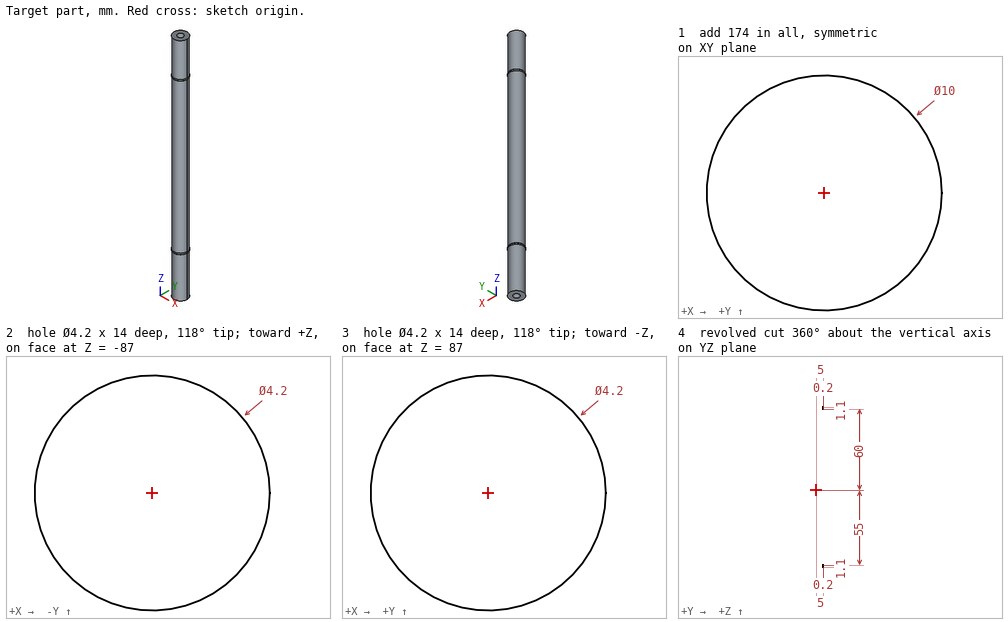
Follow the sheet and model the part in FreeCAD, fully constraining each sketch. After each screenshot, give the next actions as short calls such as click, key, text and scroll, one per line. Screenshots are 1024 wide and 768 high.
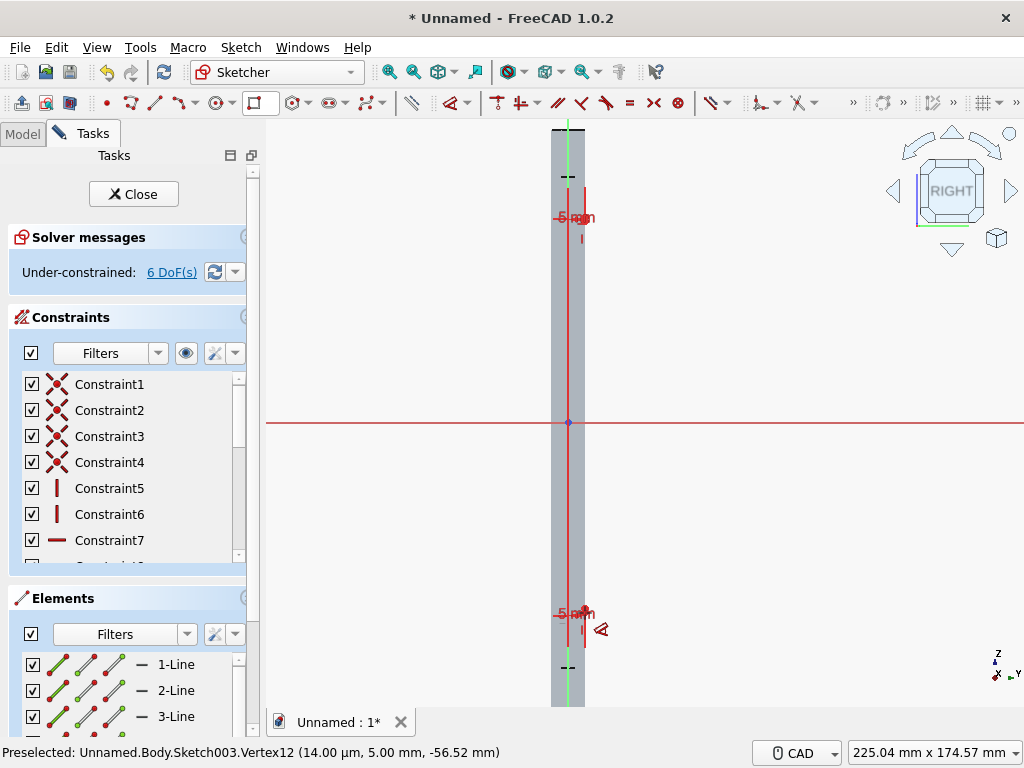
scroll(584, 219, up, 14)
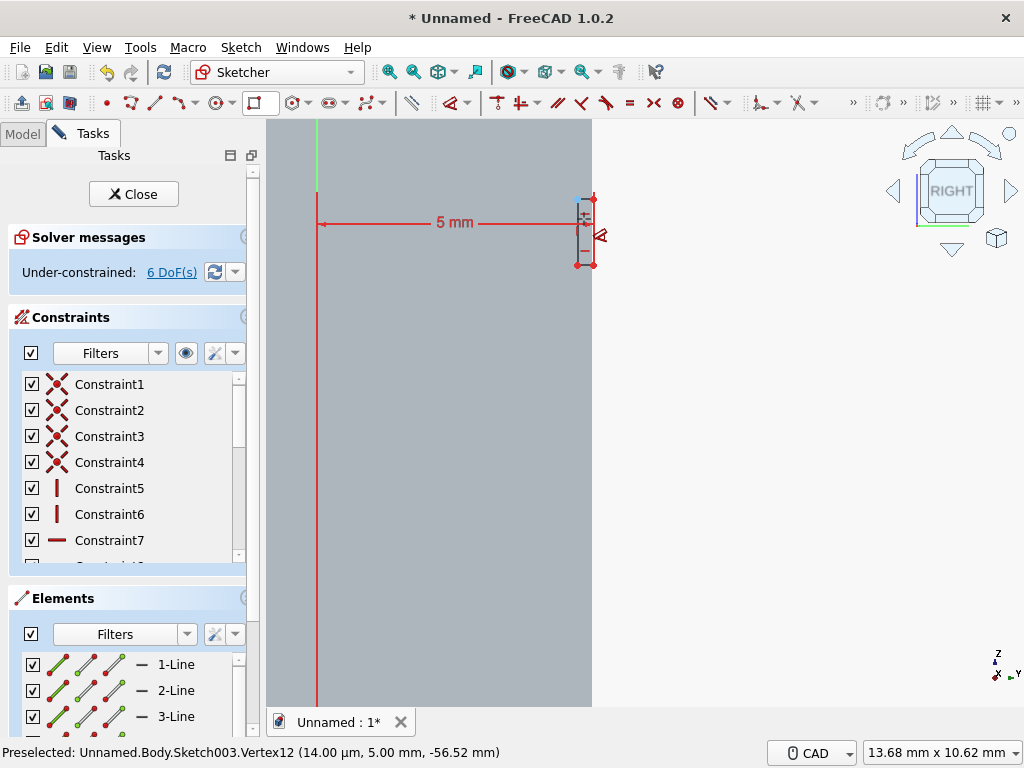
click(578, 219)
click(612, 232)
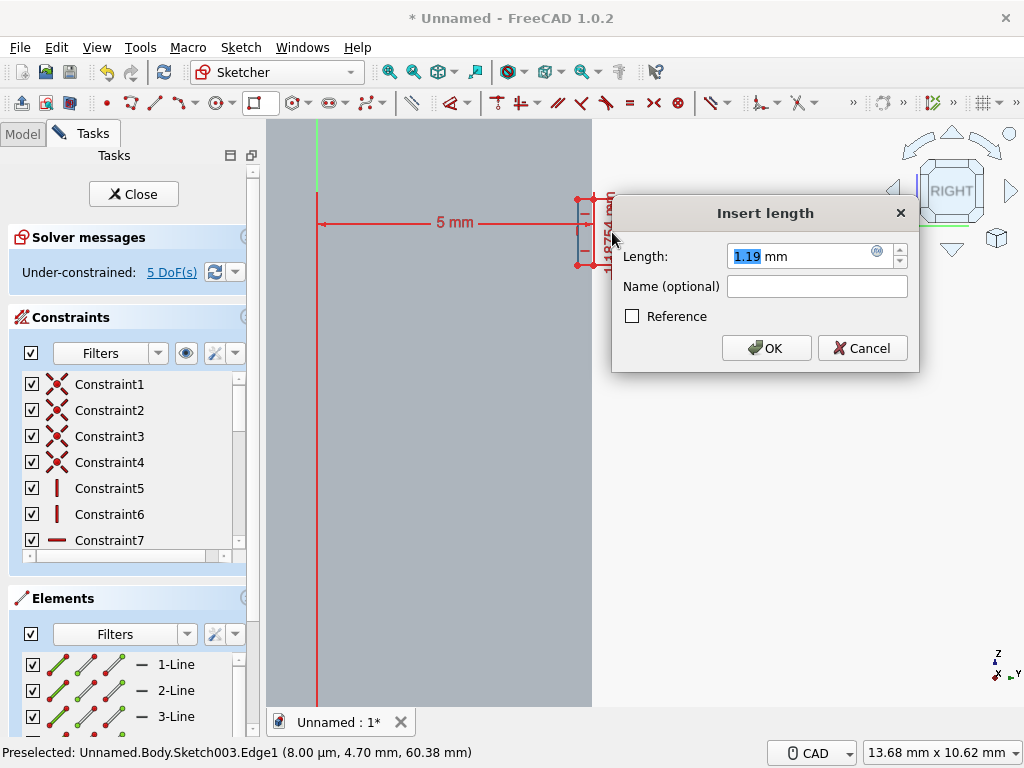
text(1.1)
key(Return)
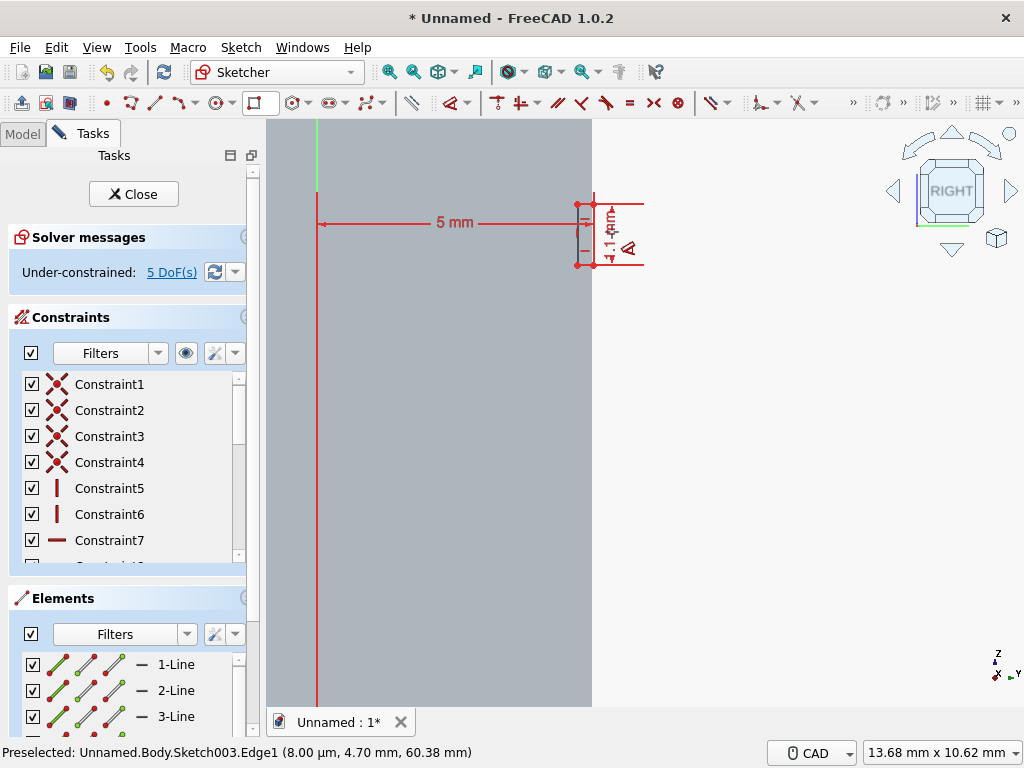
scroll(586, 265, up, 7)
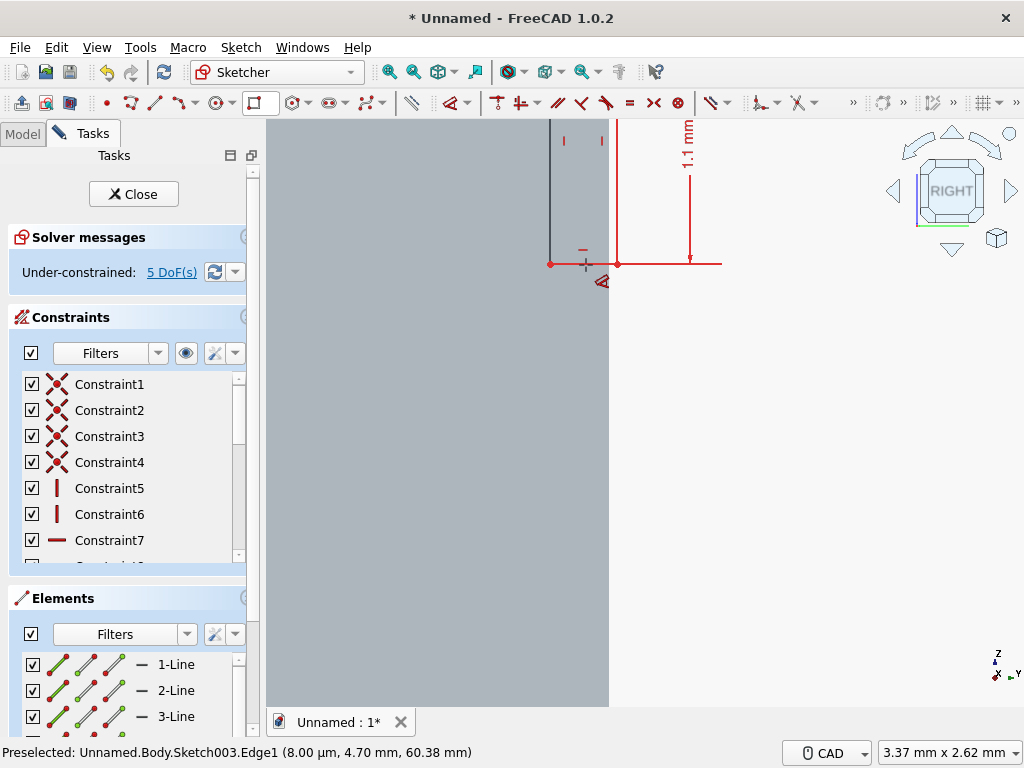
click(584, 264)
click(584, 230)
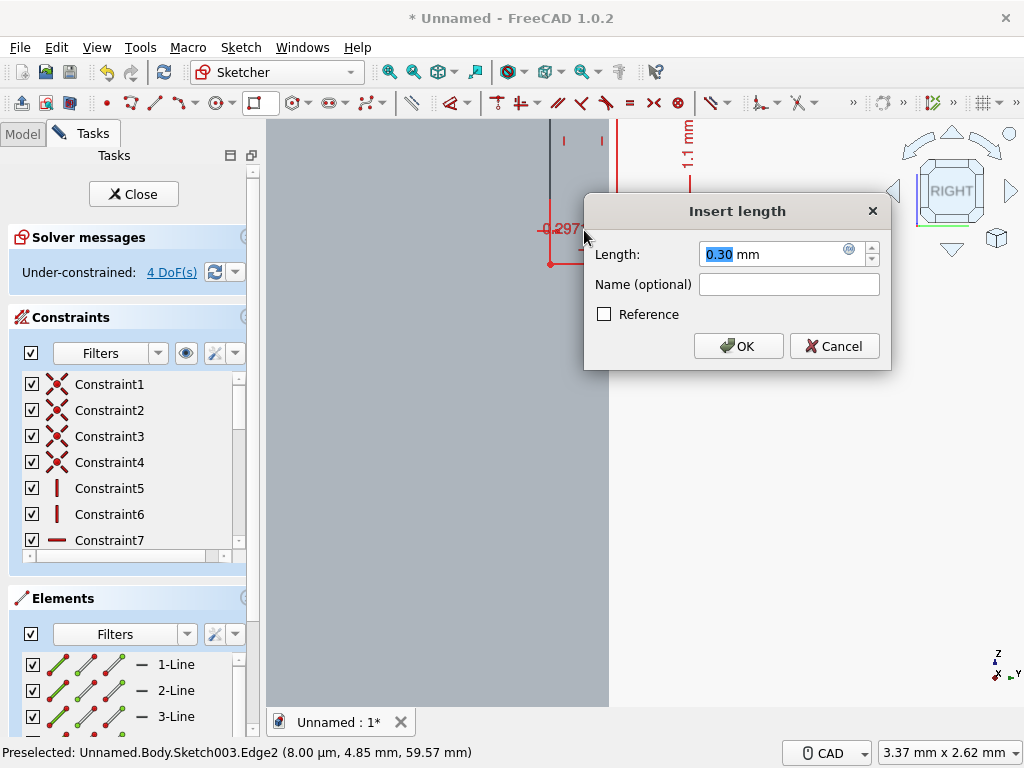
text(0.2)
key(Return)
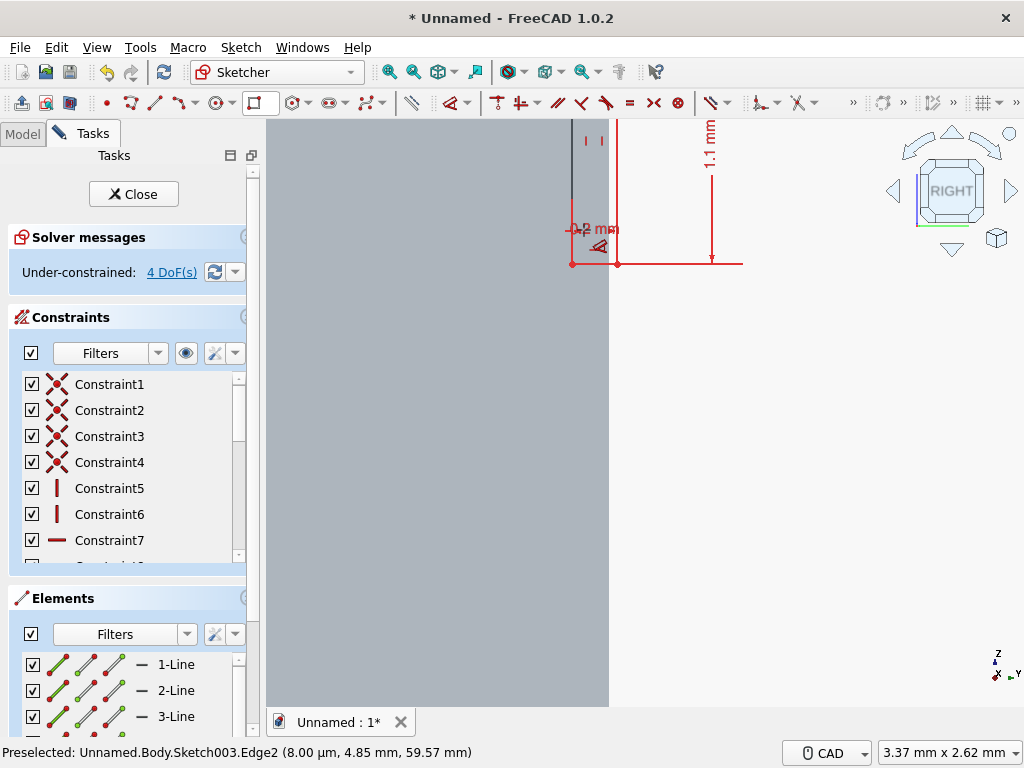
scroll(576, 413, down, 15)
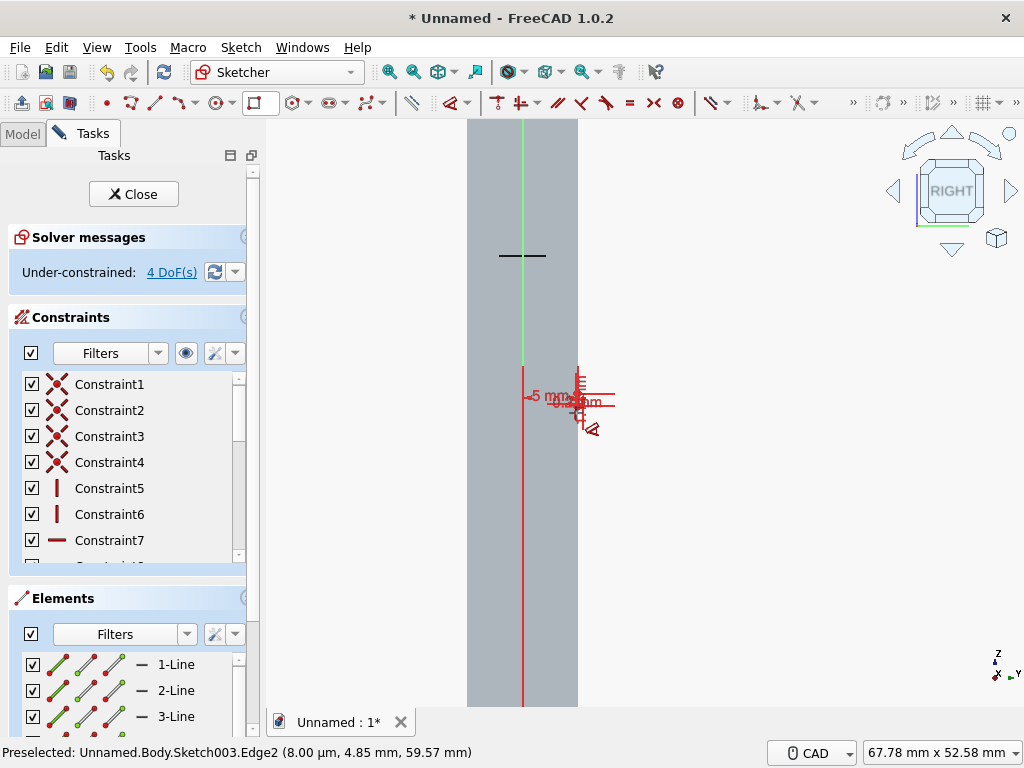
scroll(588, 147, down, 6)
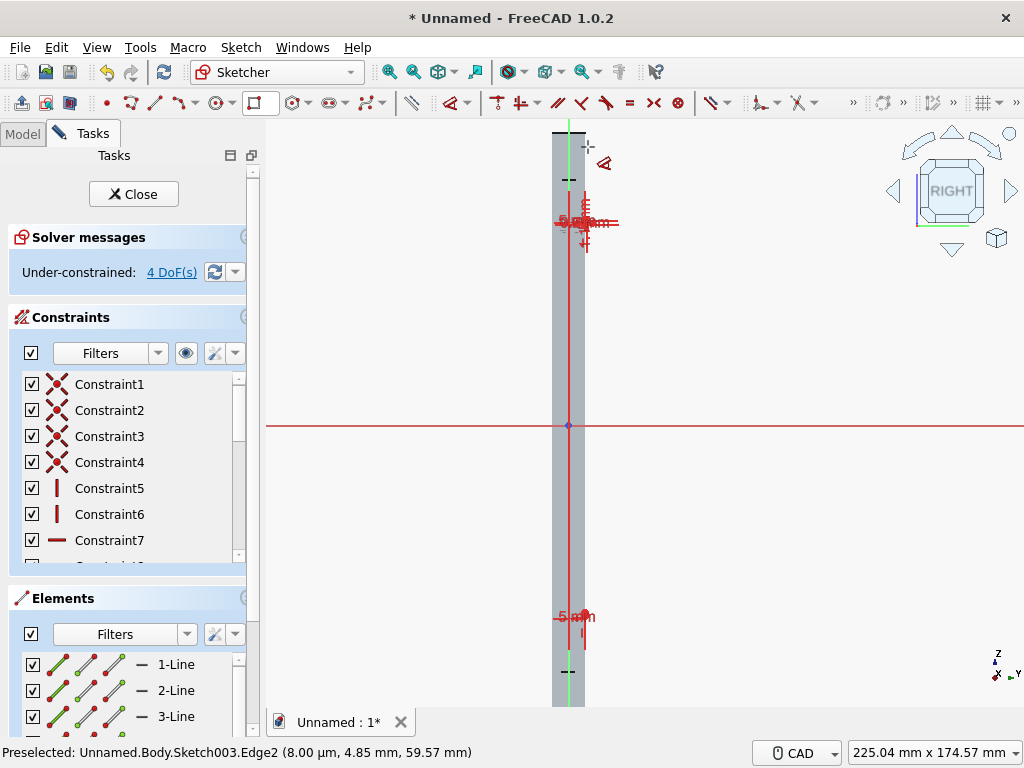
scroll(584, 613, up, 14)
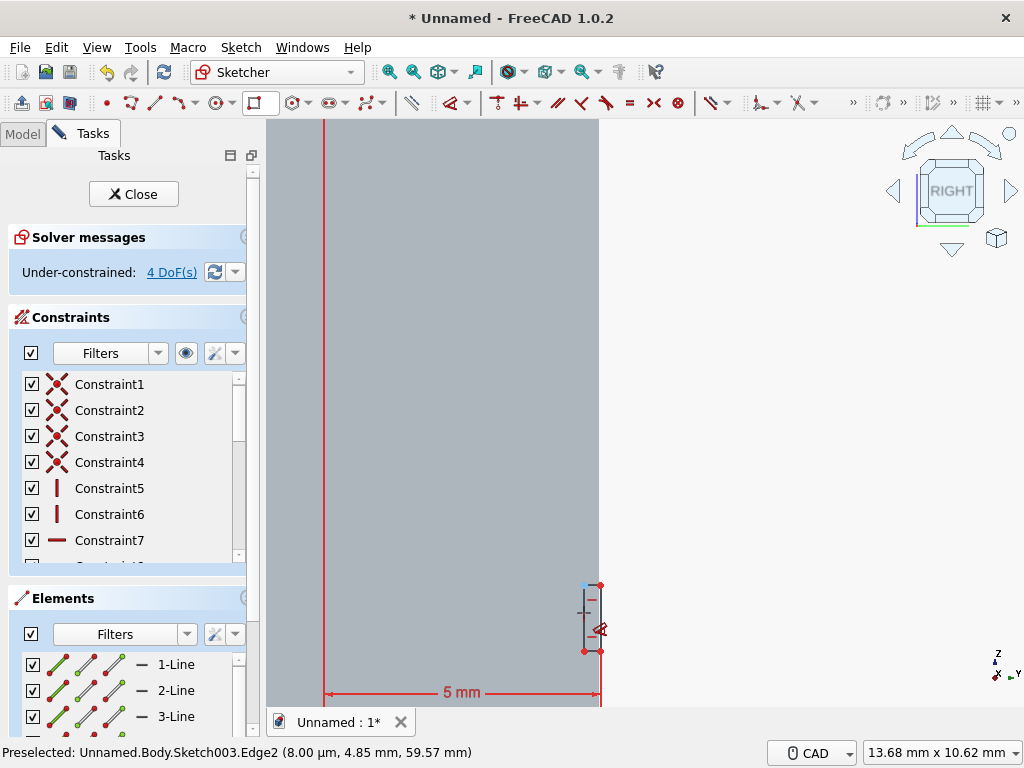
click(584, 605)
click(618, 618)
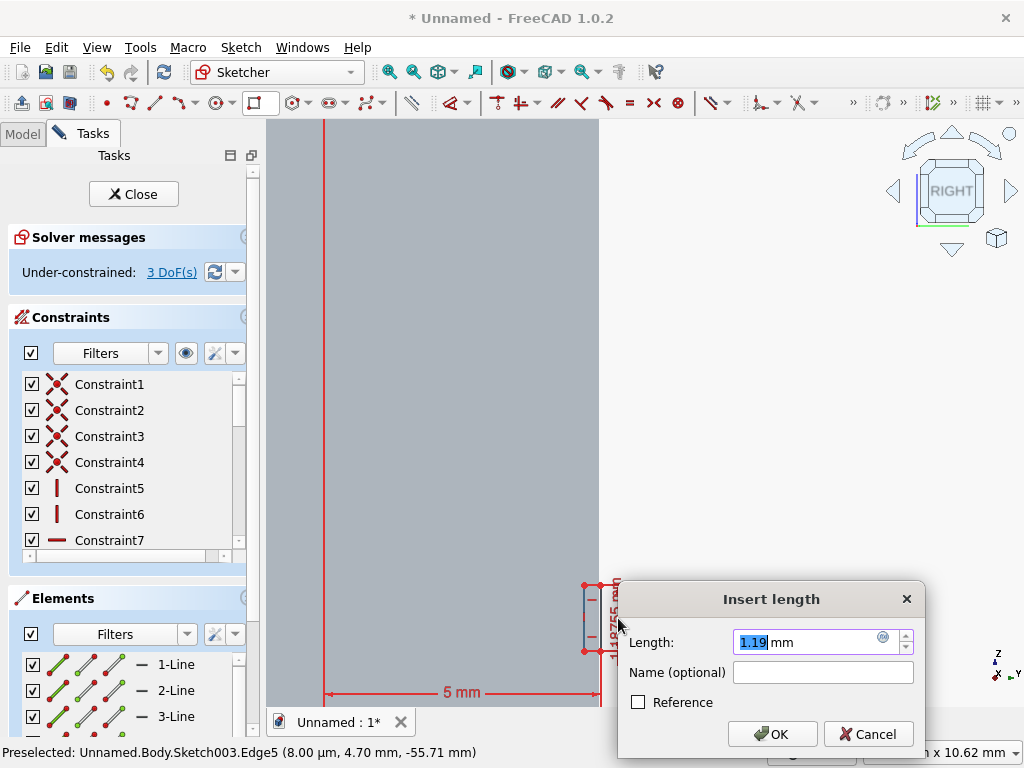
text(1.1)
key(Return)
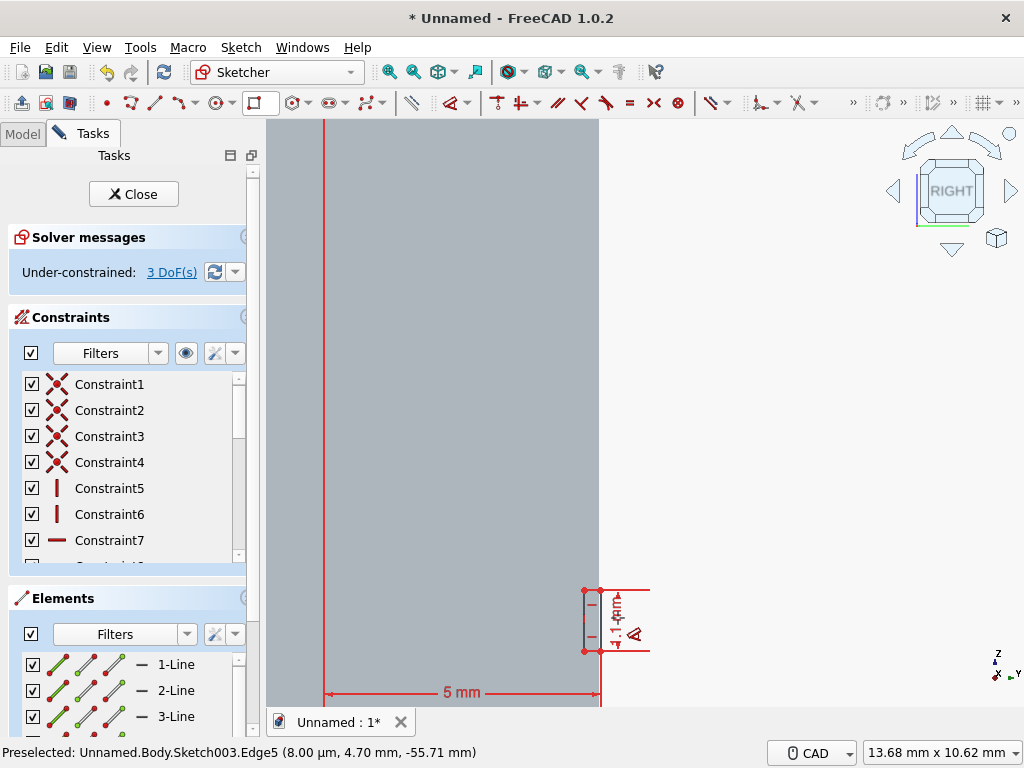
scroll(593, 651, up, 7)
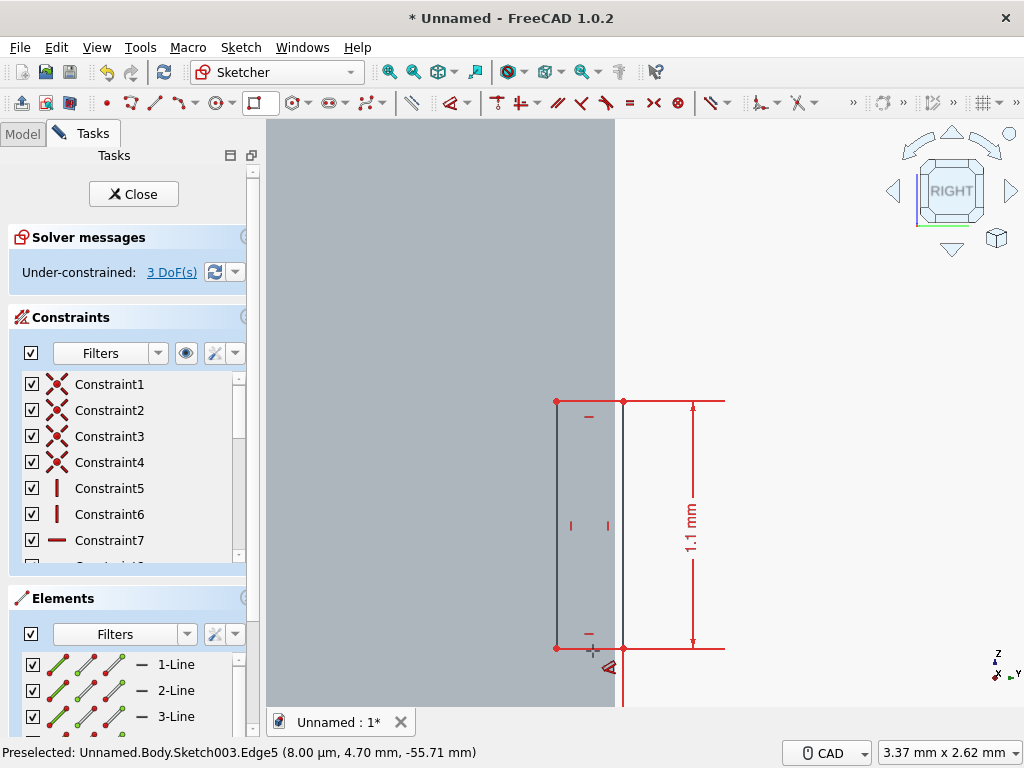
click(590, 649)
click(590, 615)